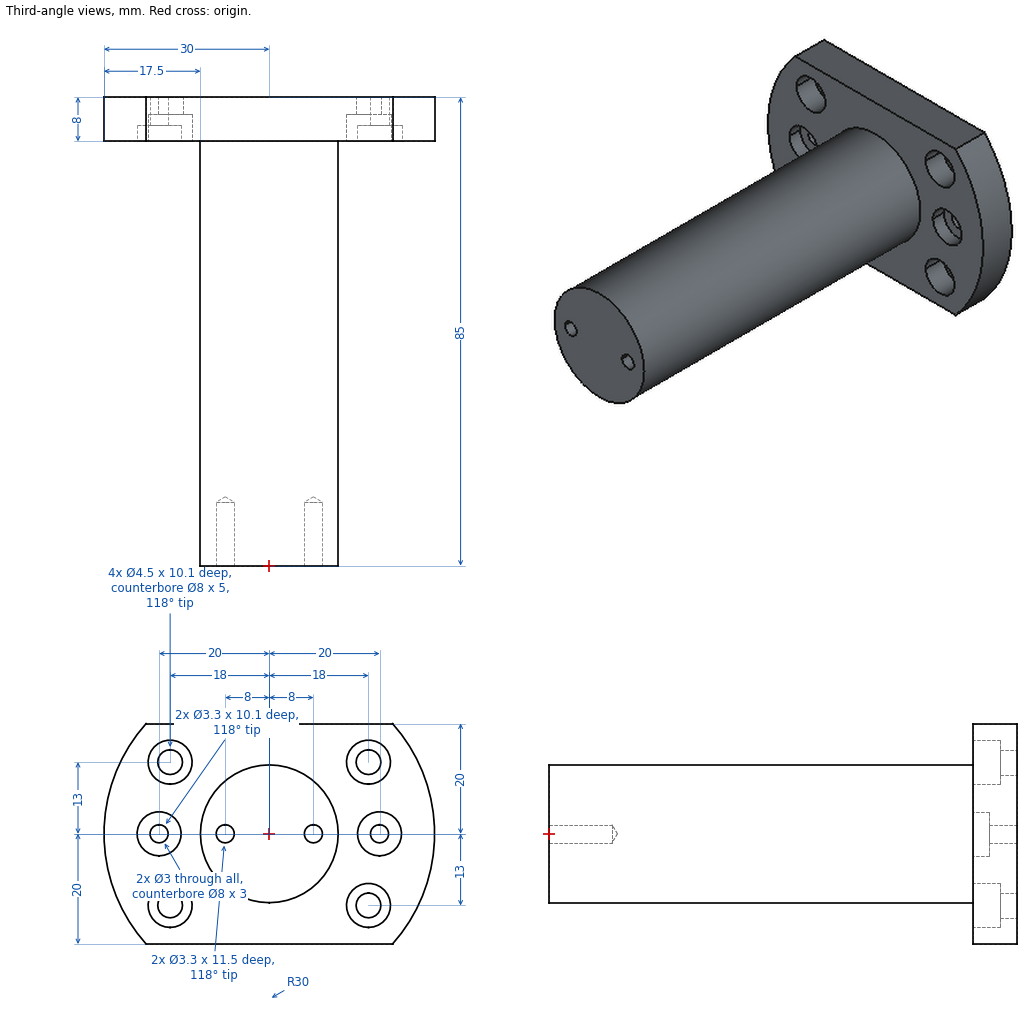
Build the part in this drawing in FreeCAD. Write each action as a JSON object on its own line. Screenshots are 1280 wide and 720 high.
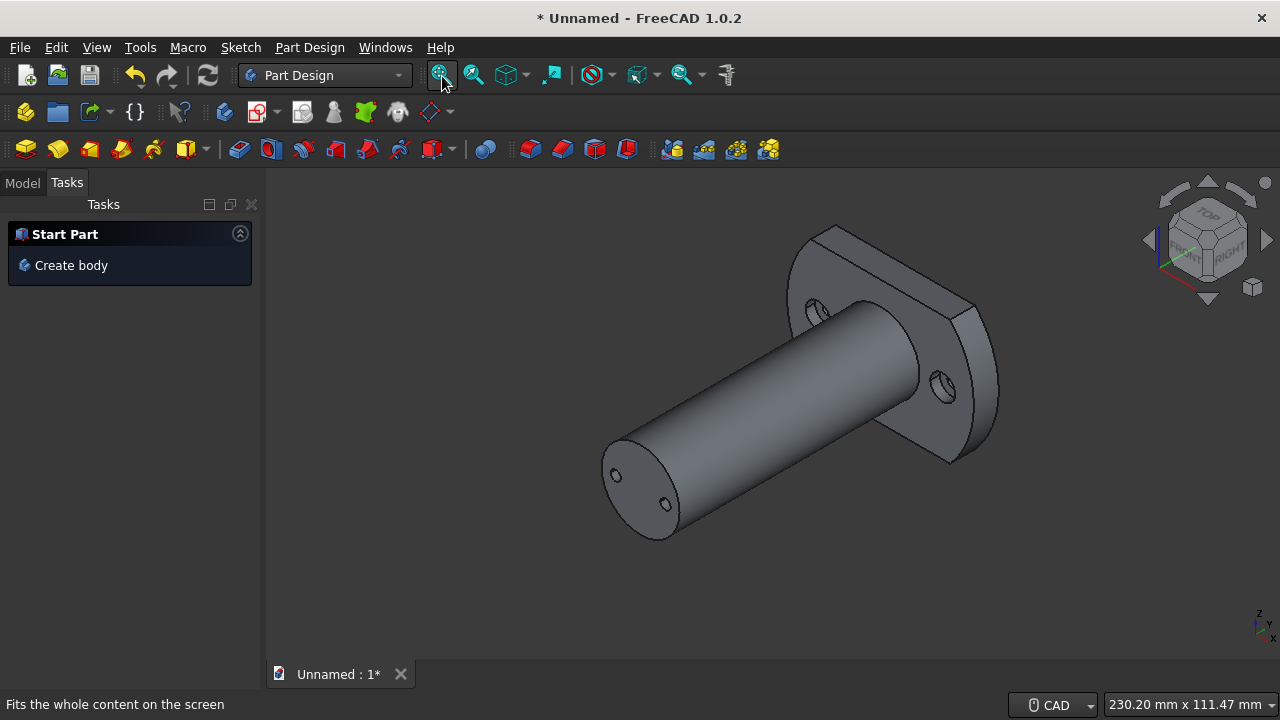
{"action": "key", "text": "1"}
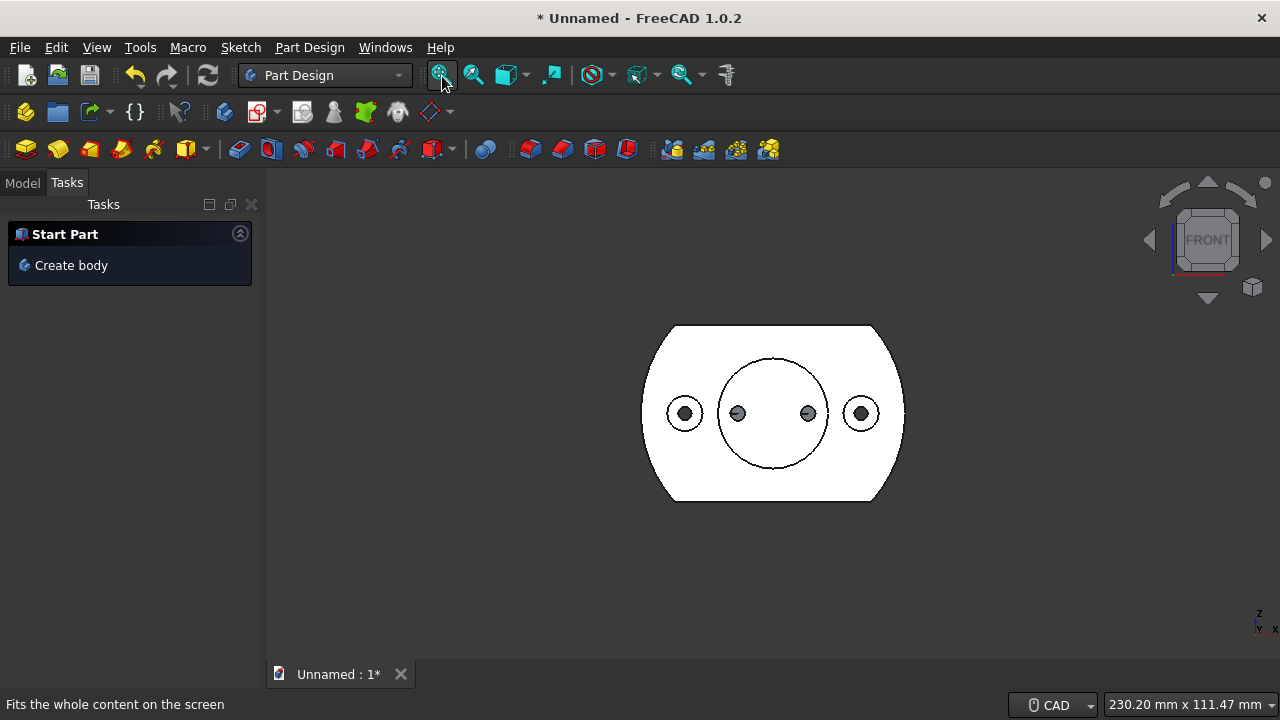
{"action": "left_click", "coordinate": [442, 76]}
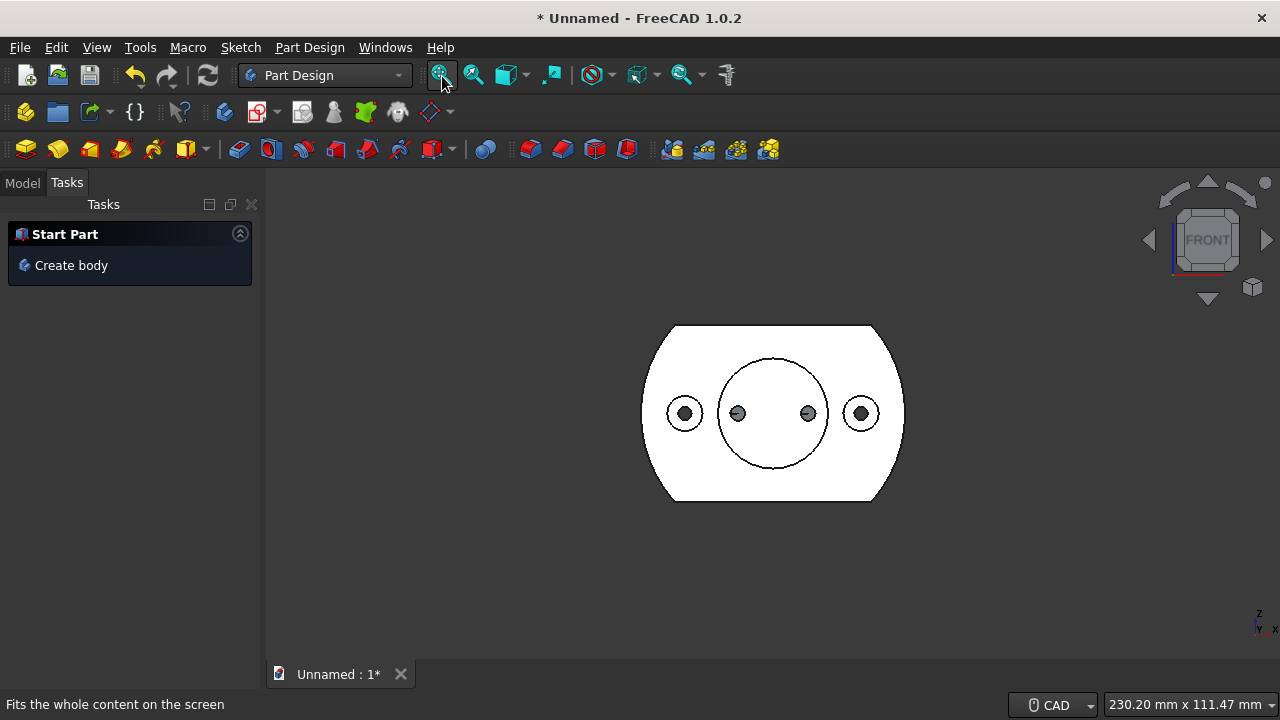
{"action": "scroll", "coordinate": [695, 407], "scroll_direction": "up", "scroll_amount": 5}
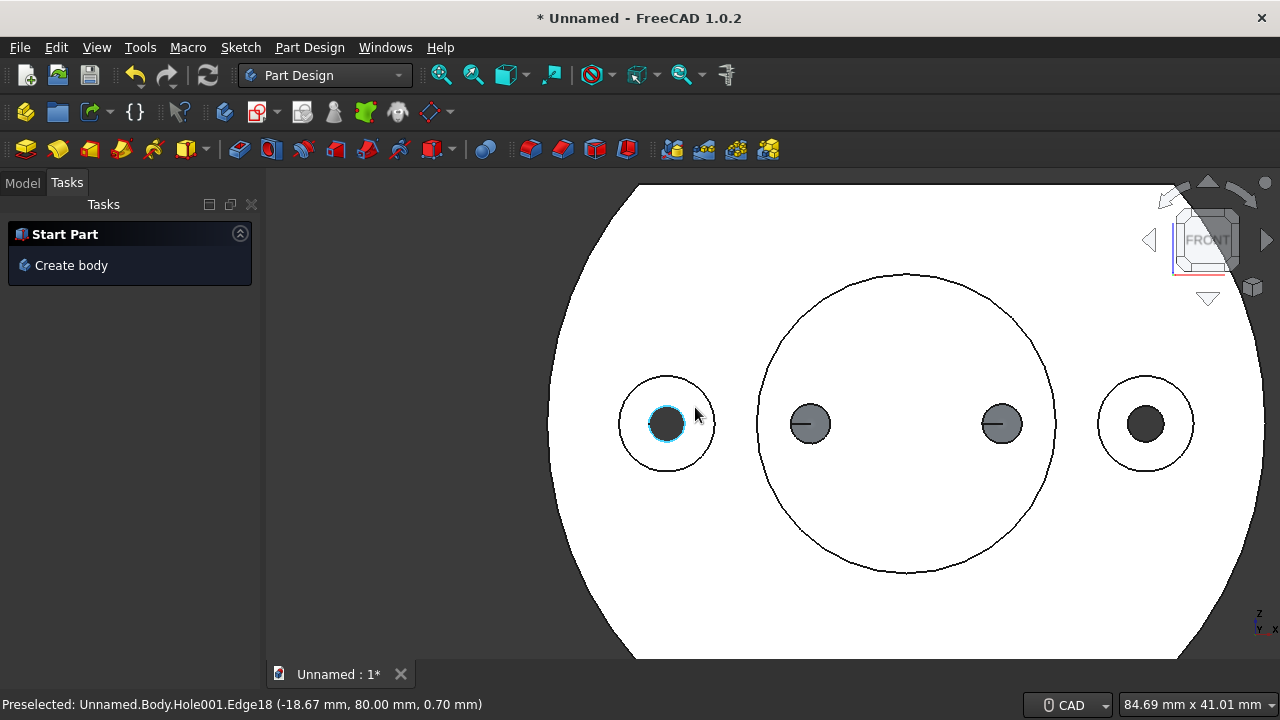
{"action": "left_click", "coordinate": [694, 409]}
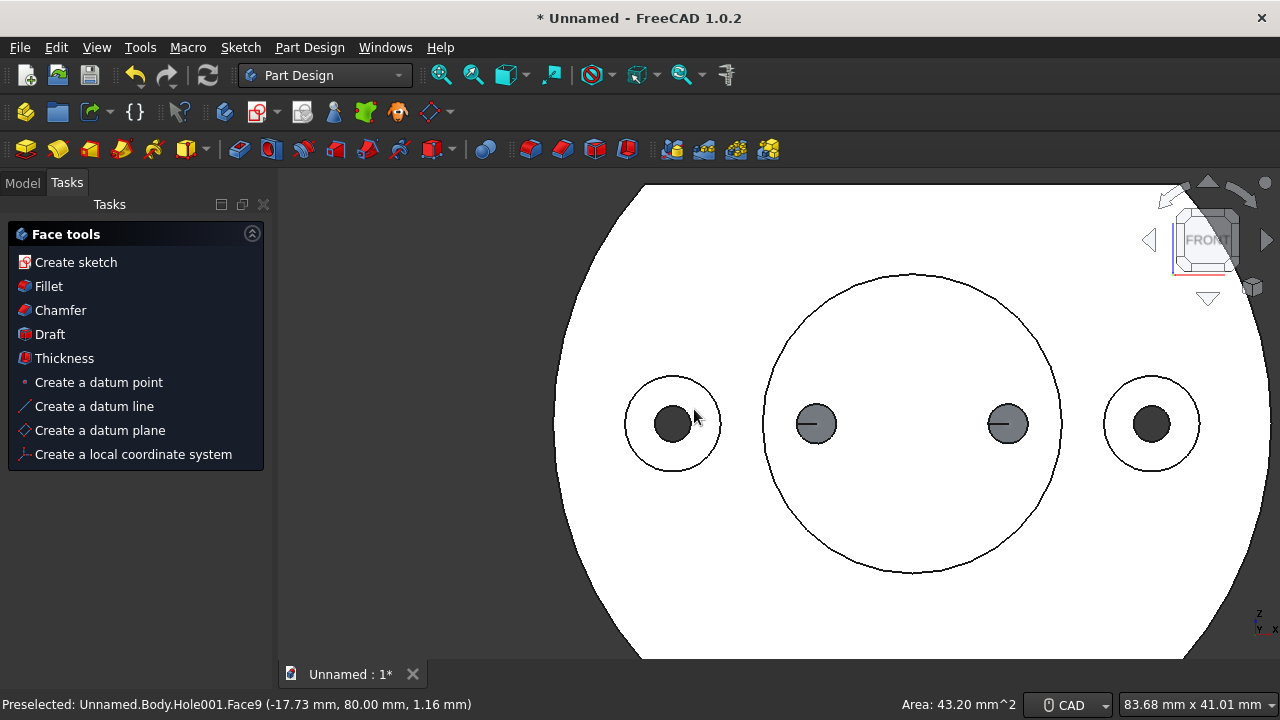
{"action": "left_click", "coordinate": [258, 112]}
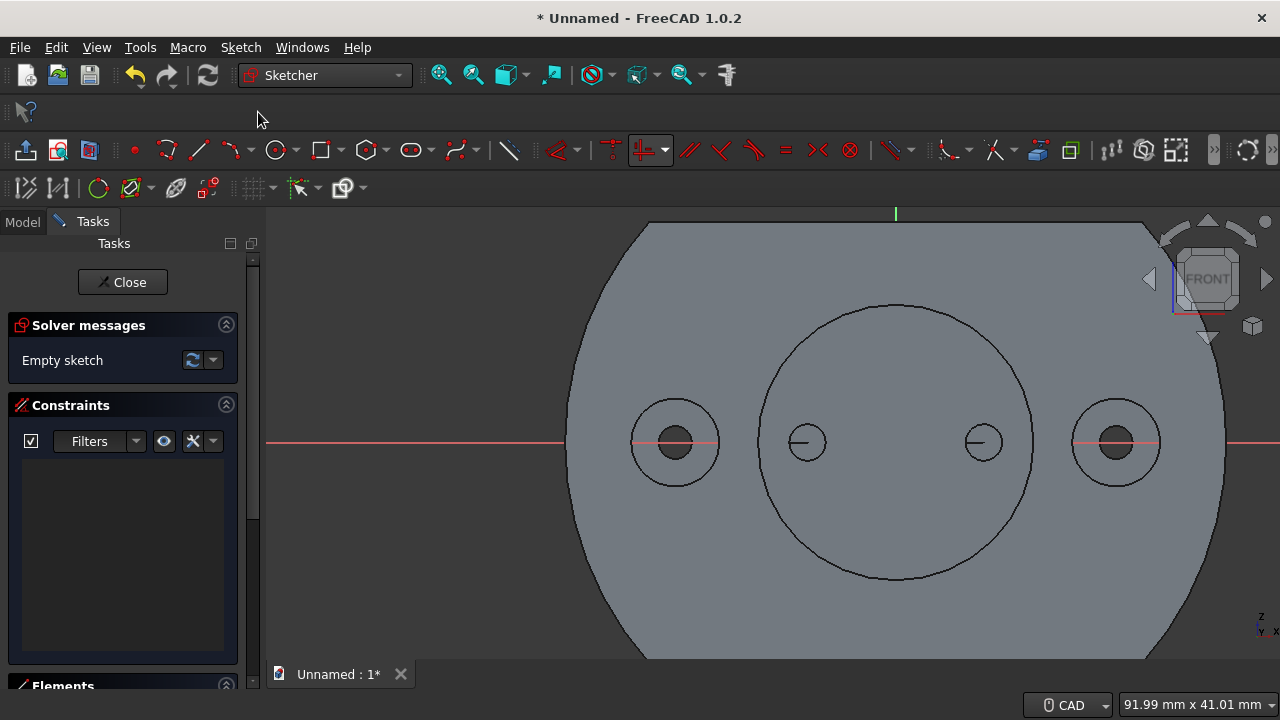
{"action": "scroll", "coordinate": [294, 390], "scroll_direction": "down", "scroll_amount": 1}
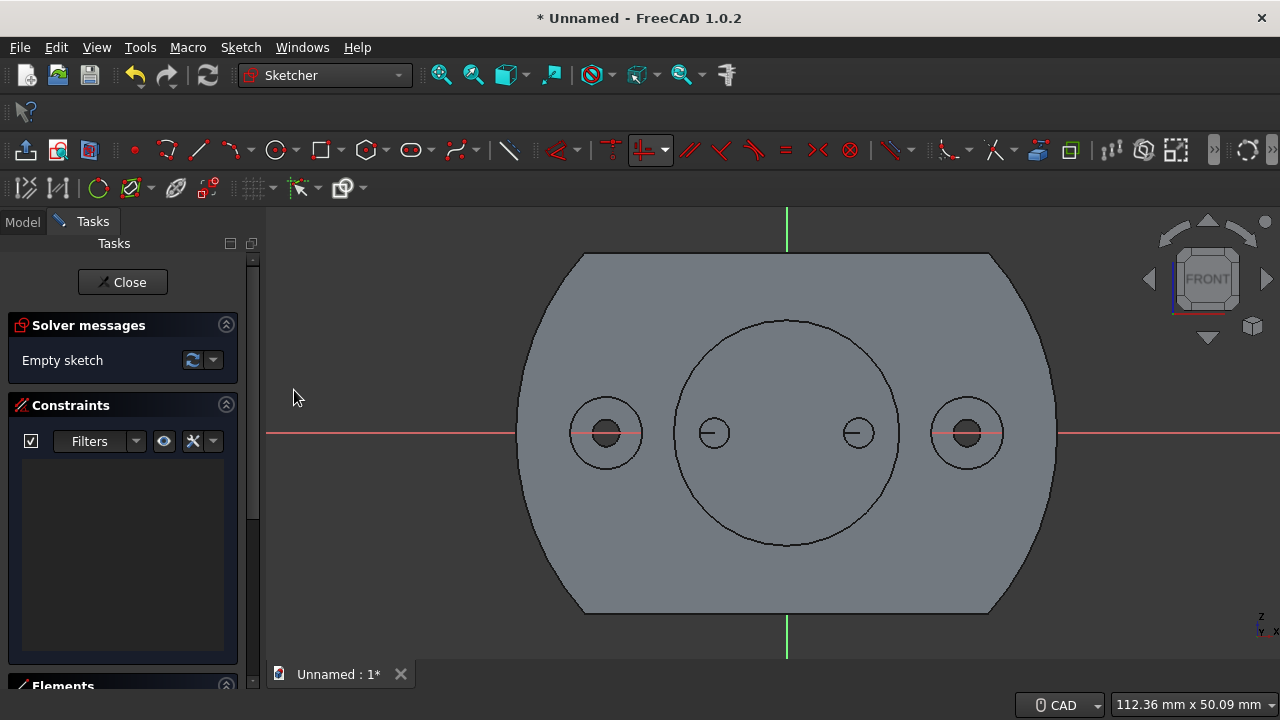
{"action": "scroll", "coordinate": [954, 433], "scroll_direction": "up", "scroll_amount": 2}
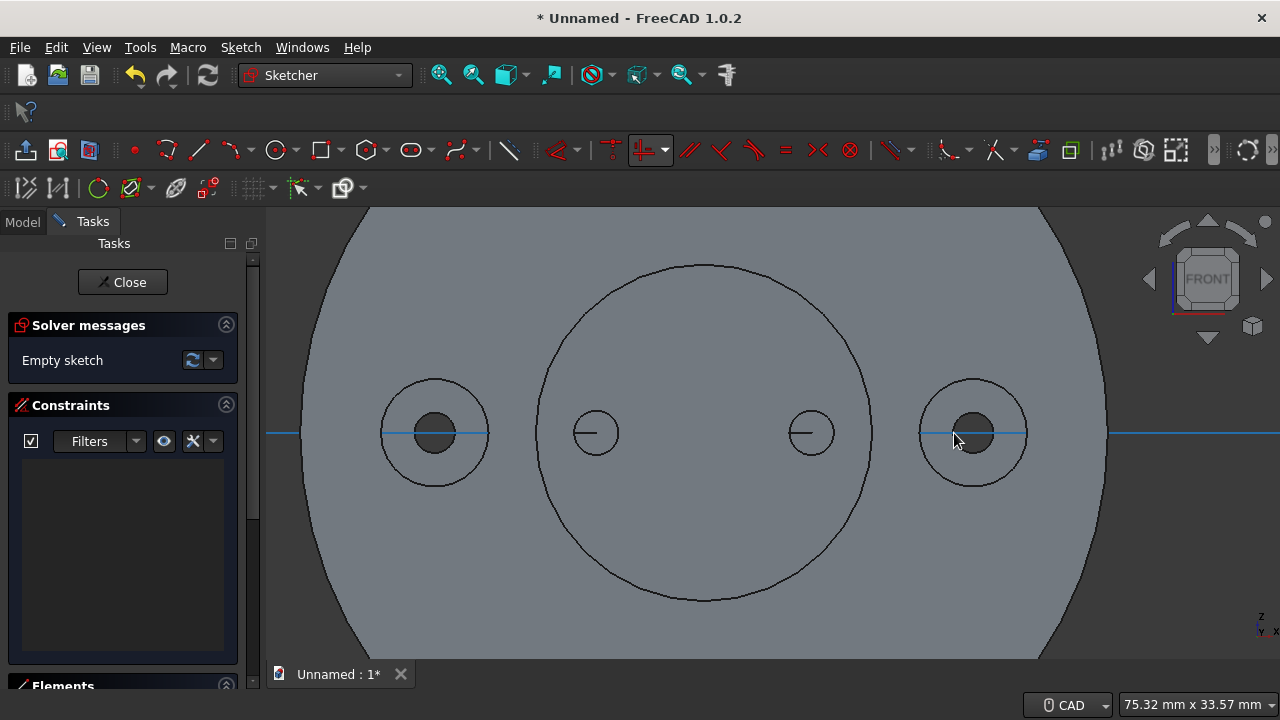
{"action": "left_click", "coordinate": [276, 150]}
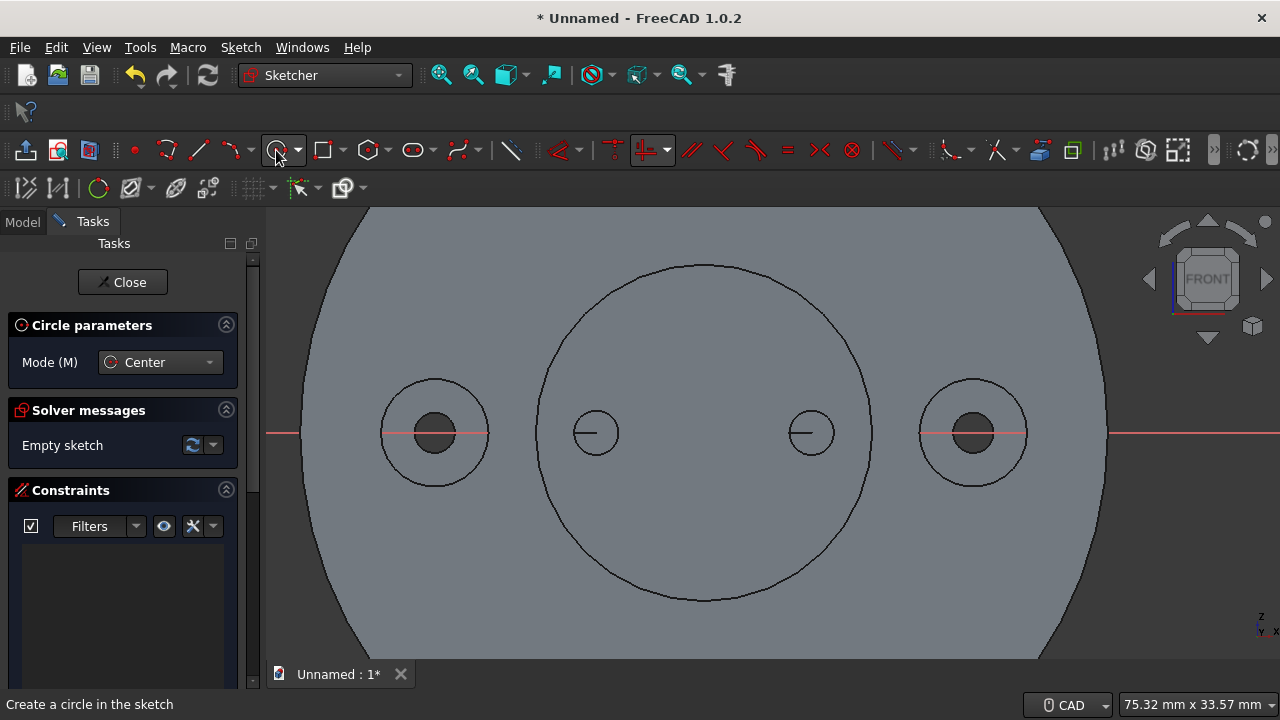
{"action": "left_click", "coordinate": [435, 433]}
{"action": "mouse_move", "coordinate": [450, 417]}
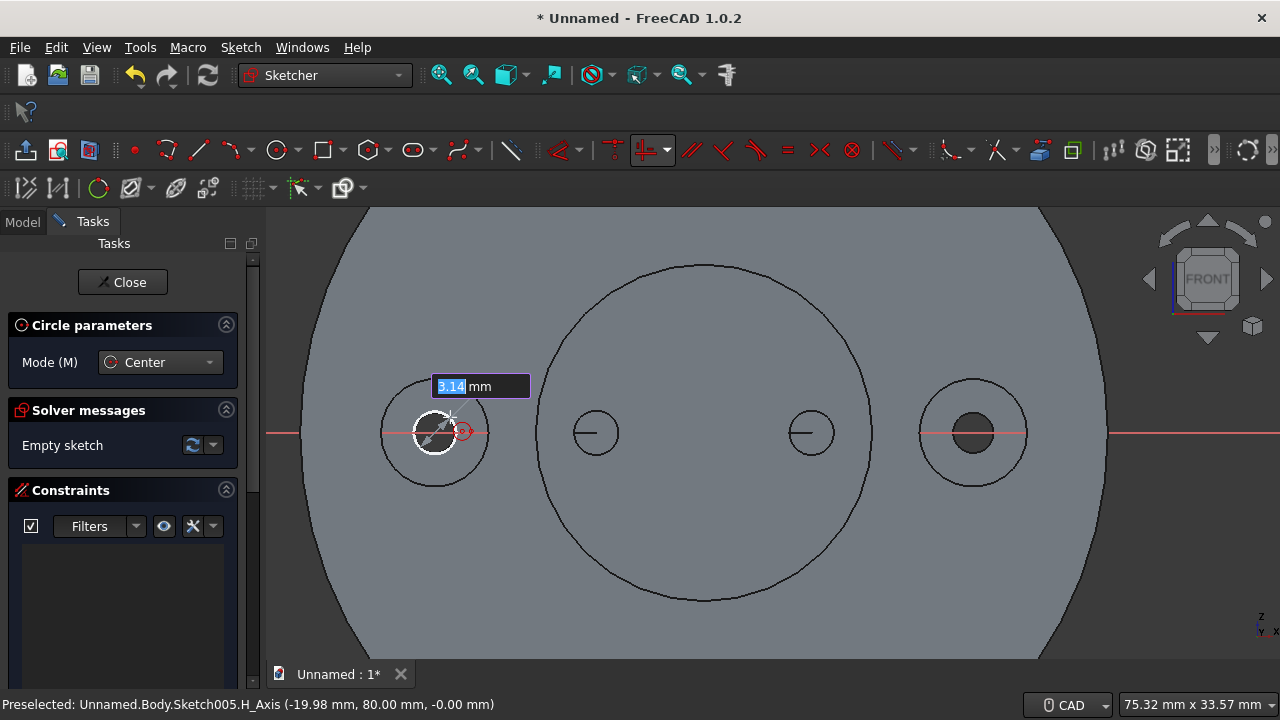
{"action": "type", "text": "3.3"}
{"action": "key", "text": "Return"}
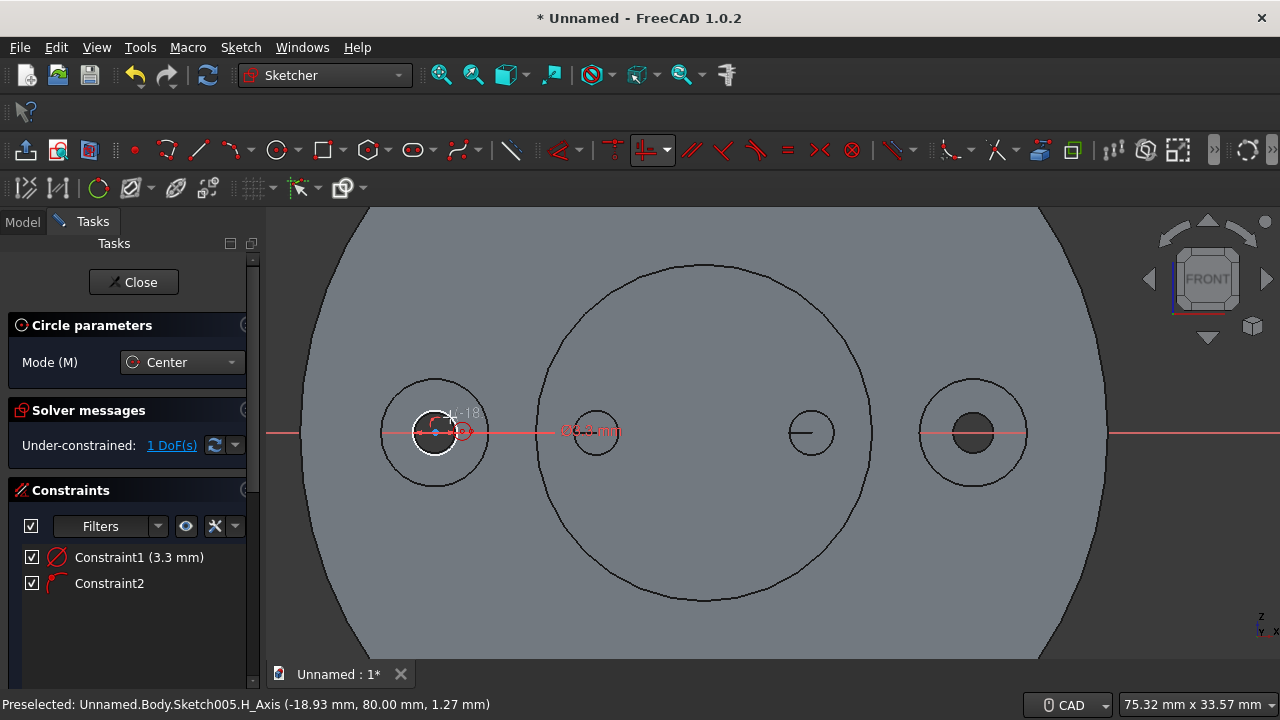
{"action": "left_click", "coordinate": [973, 433]}
{"action": "mouse_move", "coordinate": [989, 417]}